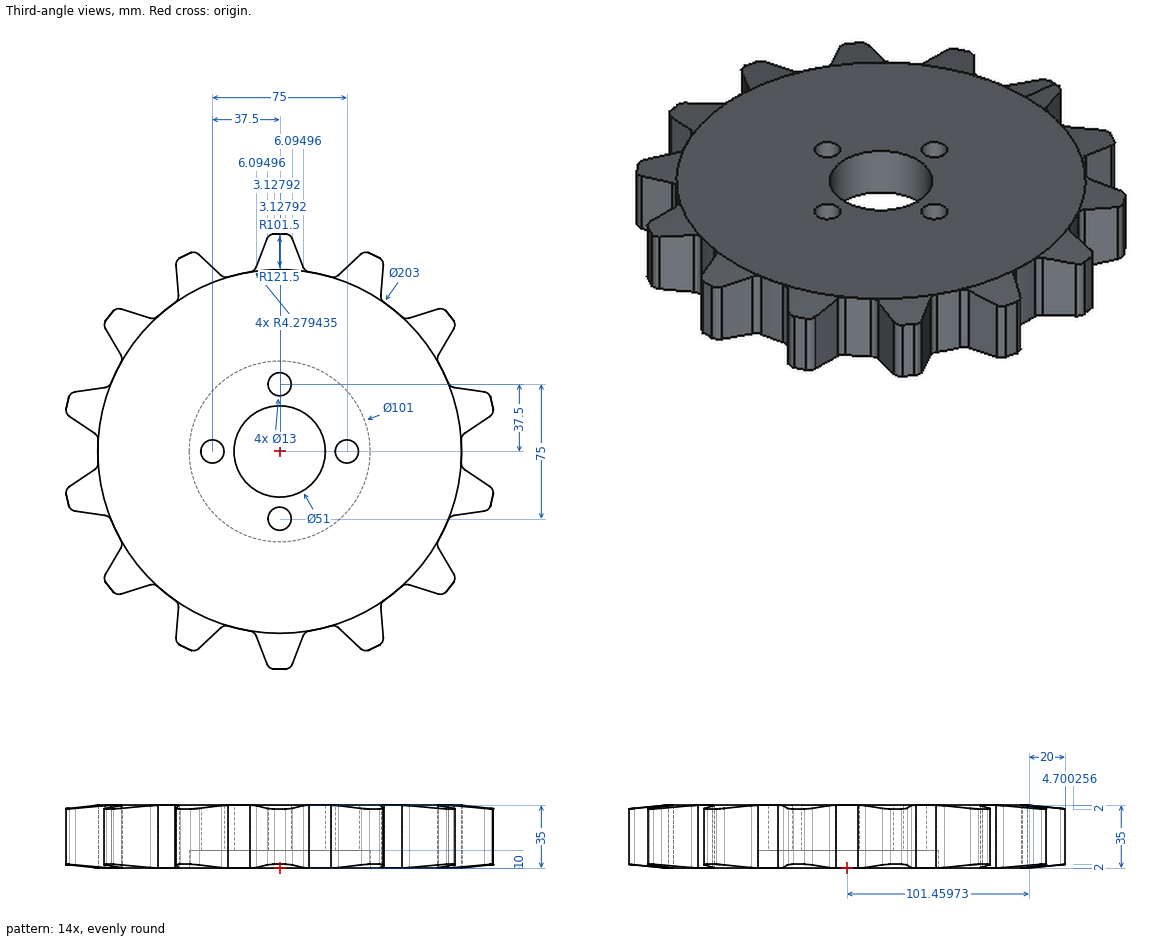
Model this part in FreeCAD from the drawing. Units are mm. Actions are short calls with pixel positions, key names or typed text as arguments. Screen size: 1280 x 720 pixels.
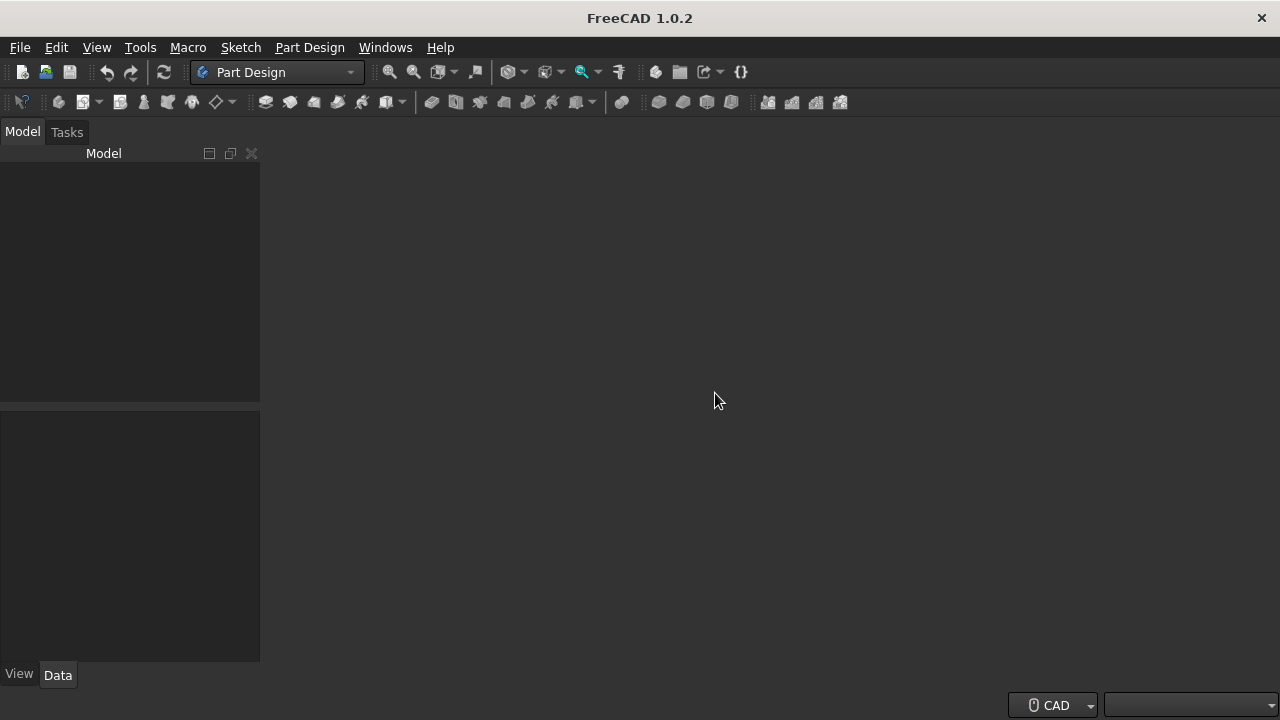
click(22, 72)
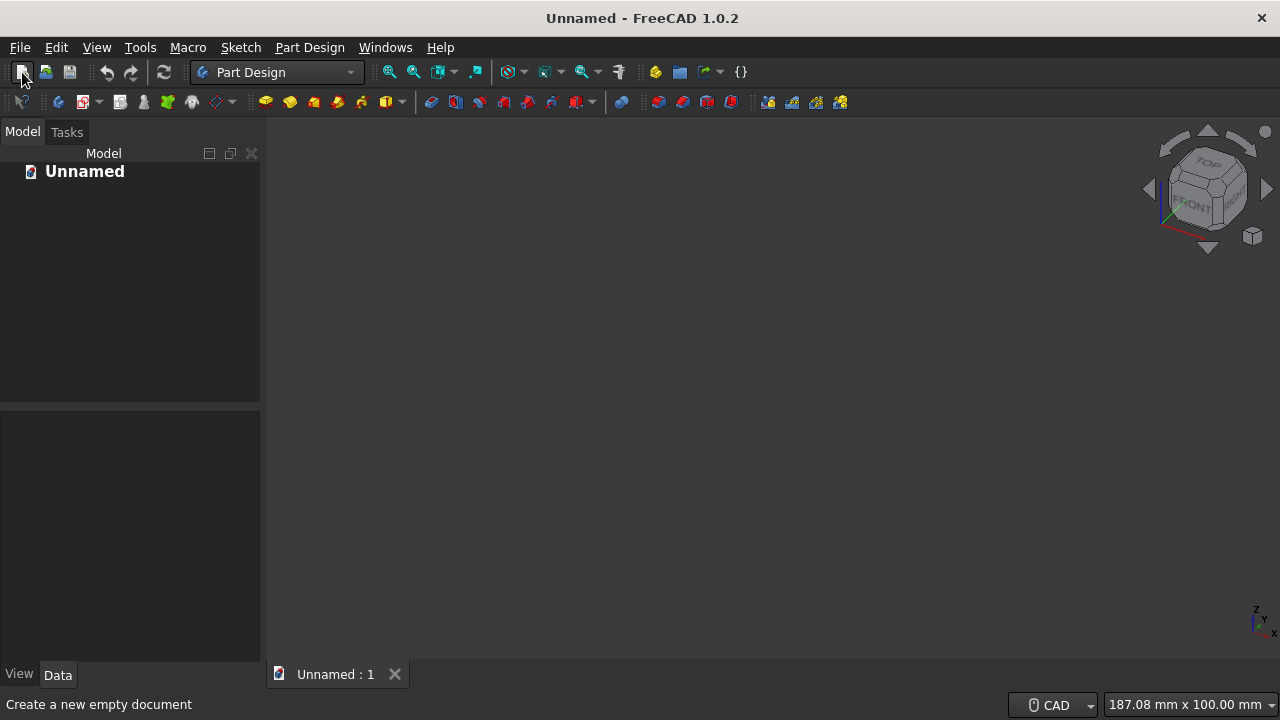
click(84, 102)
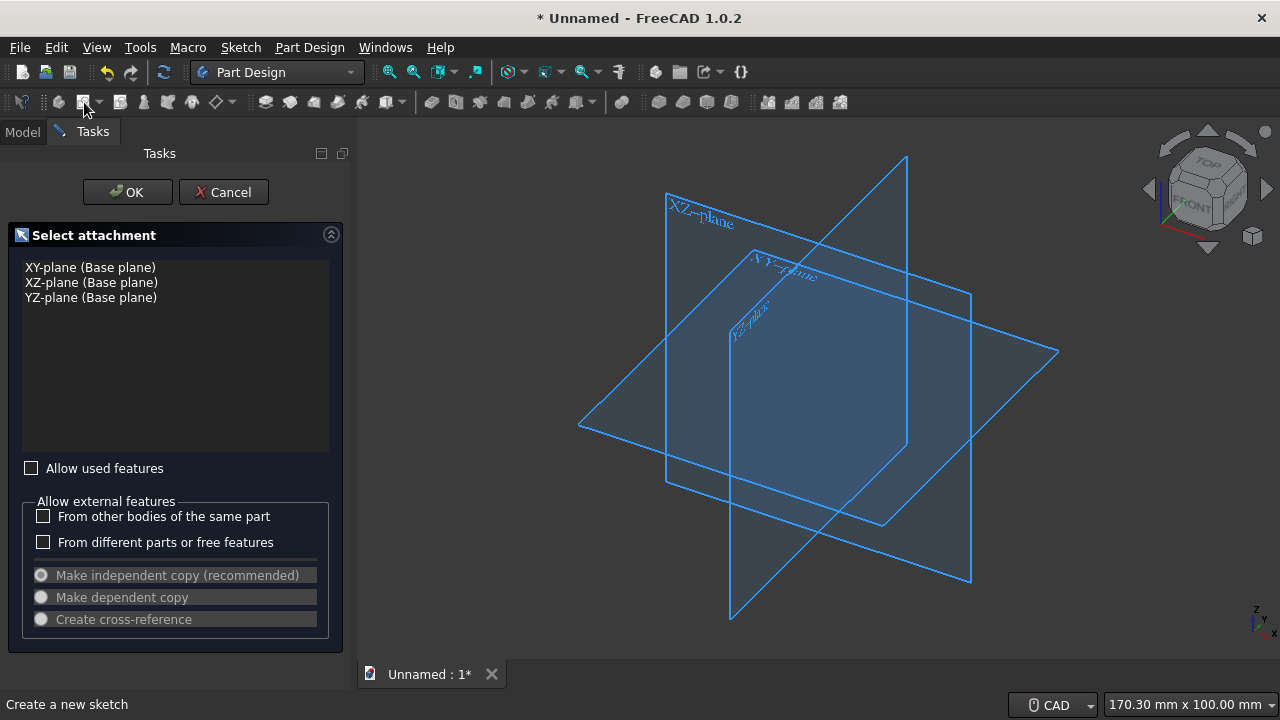
click(82, 268)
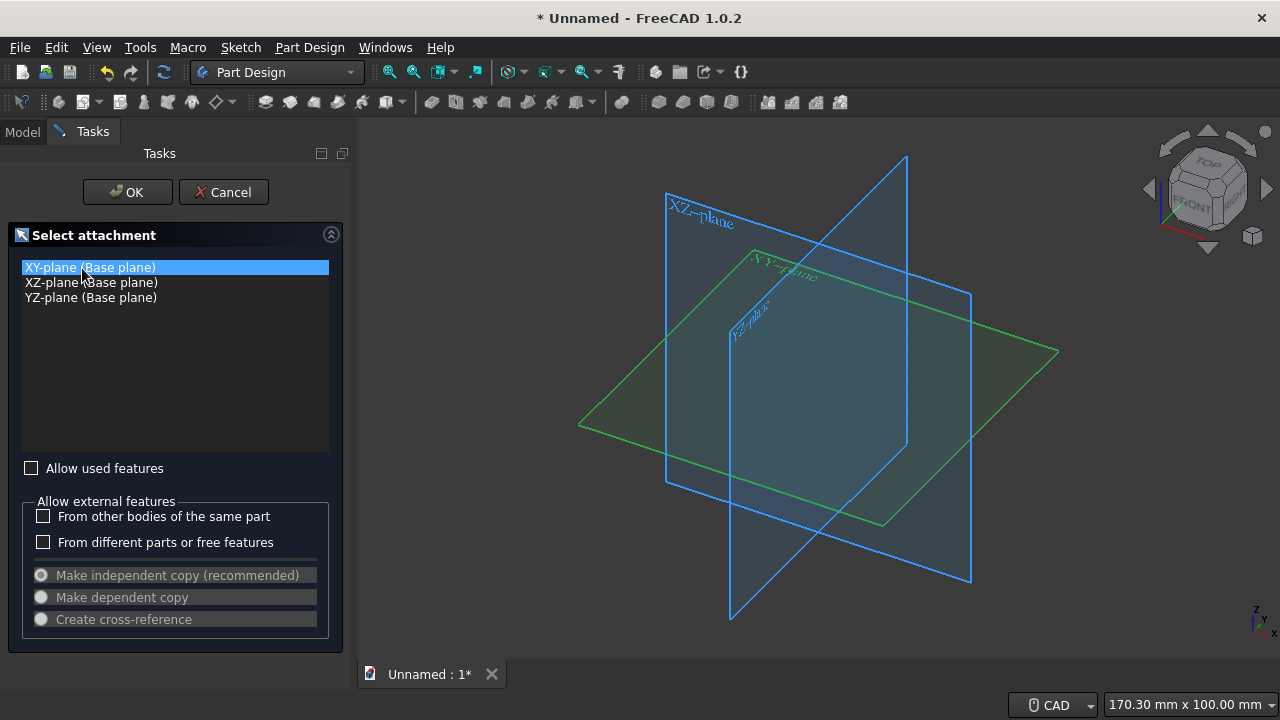
click(128, 192)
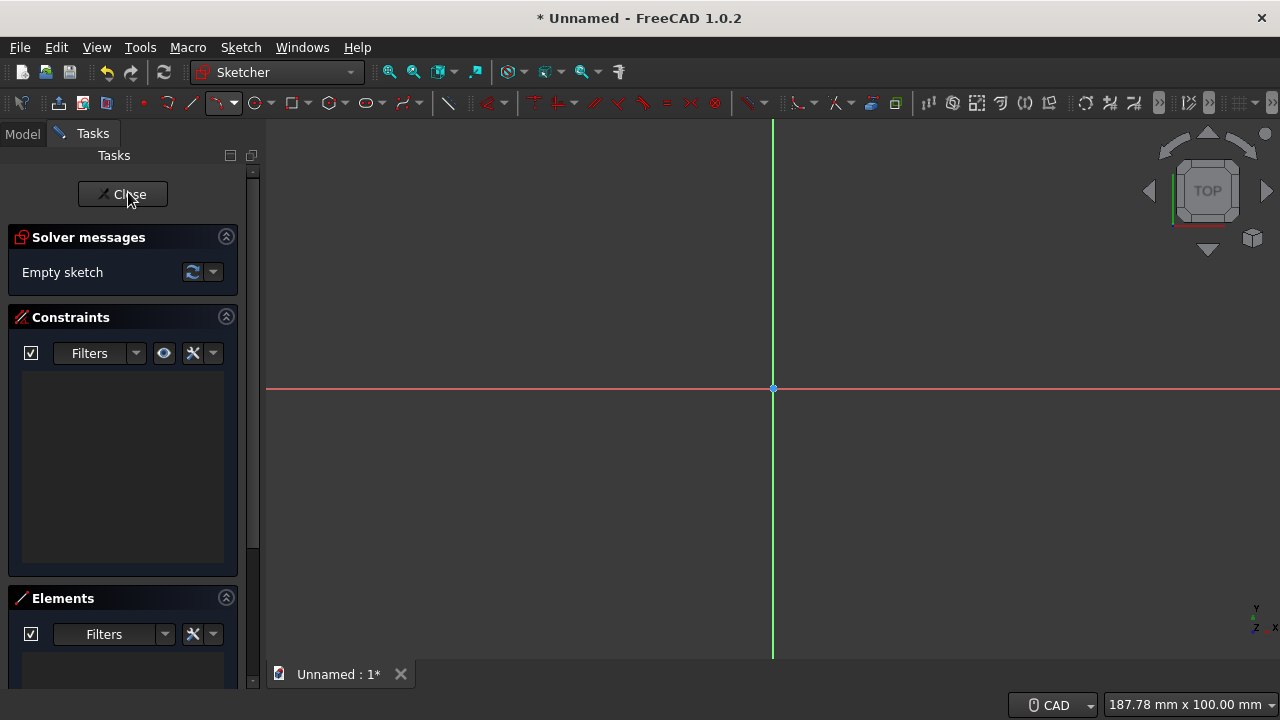
scroll(675, 389, down, 6)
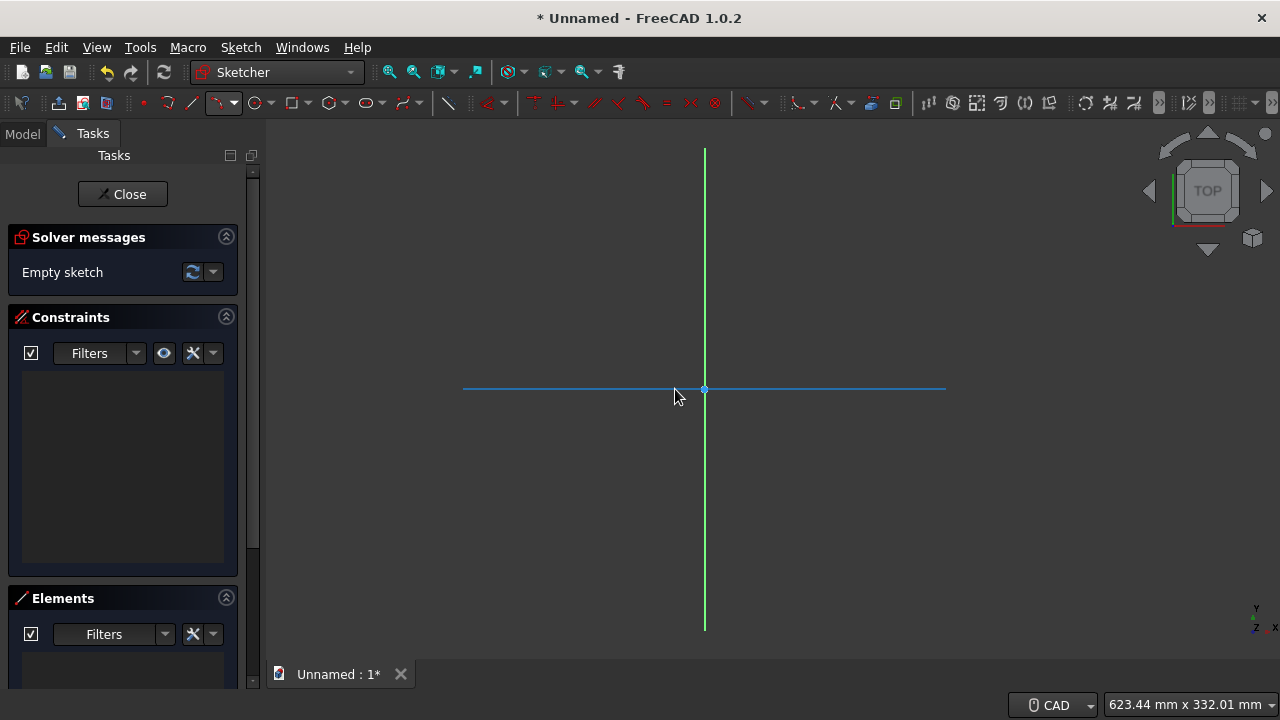
click(256, 104)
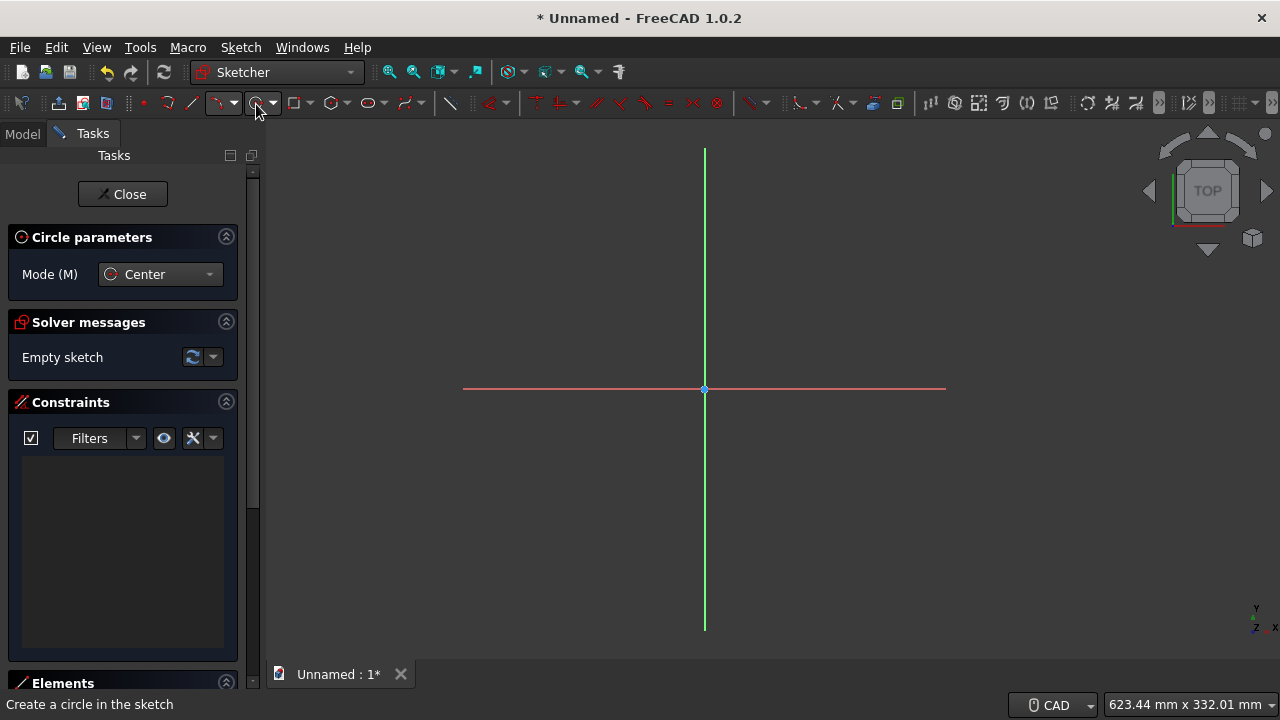
click(705, 389)
move(822, 273)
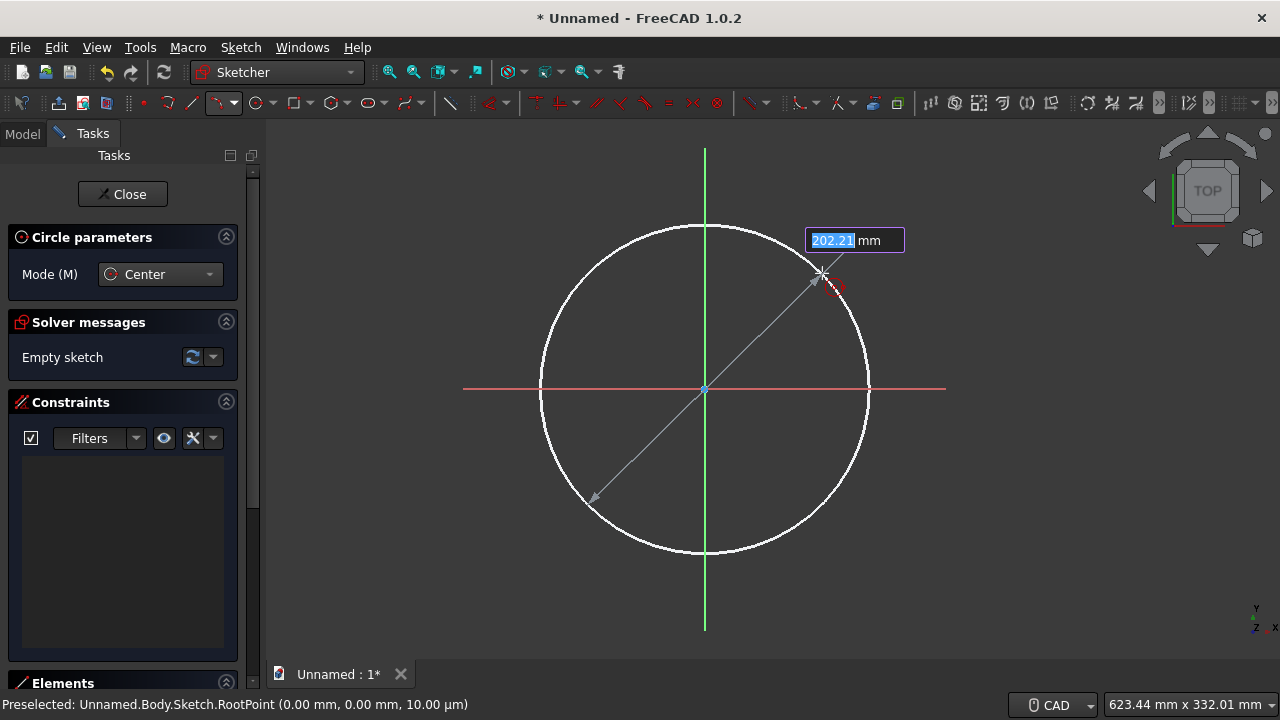
text(203)
key(Return)
key(Escape)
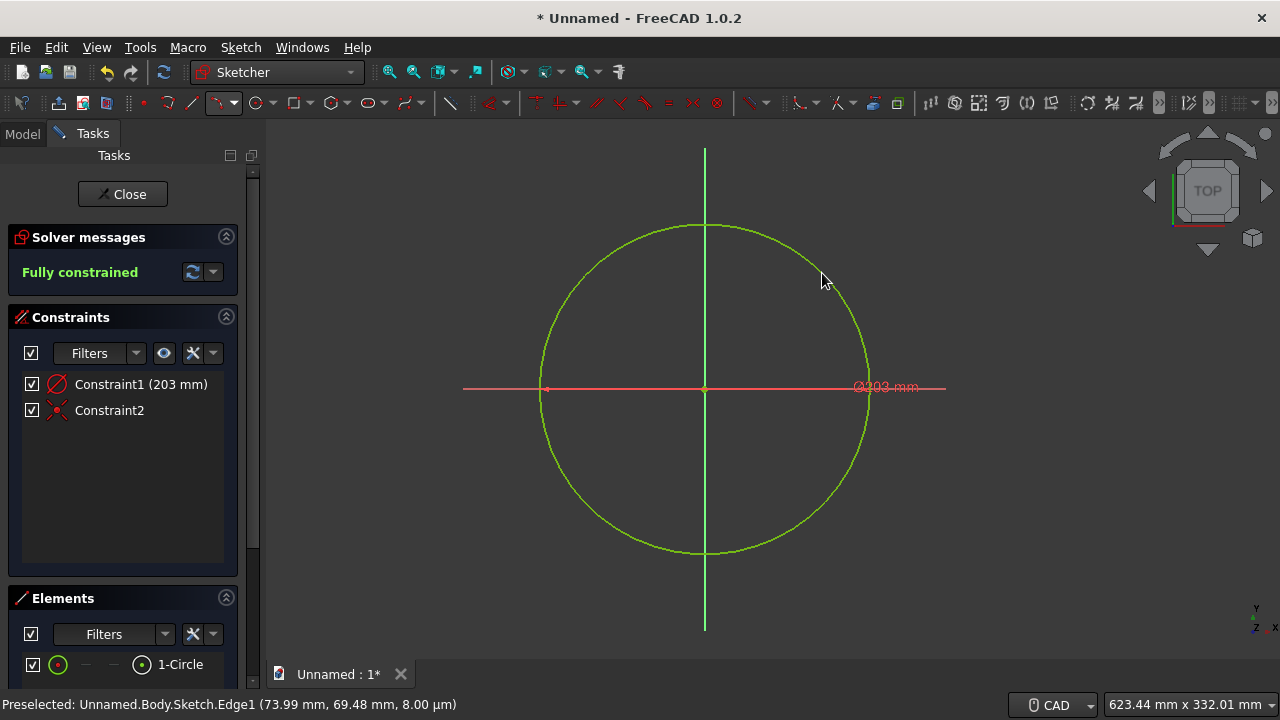
click(123, 194)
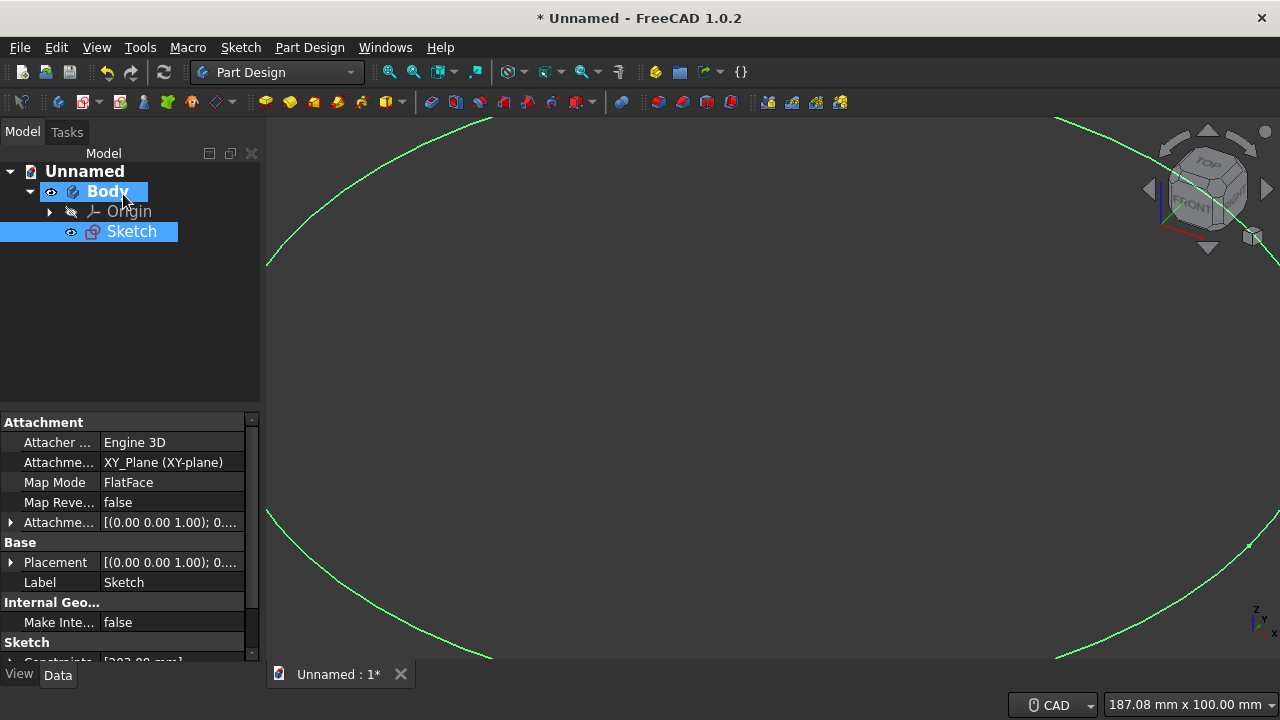
click(266, 102)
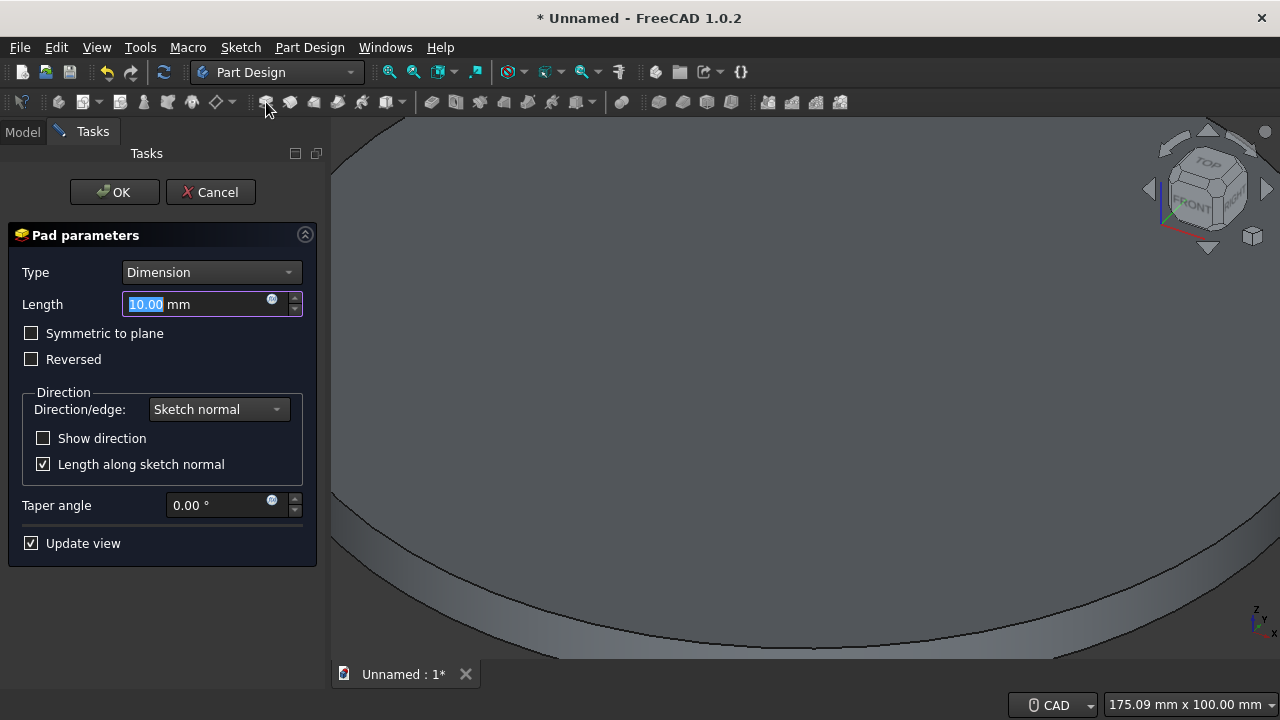
text(35)
key(Tab)